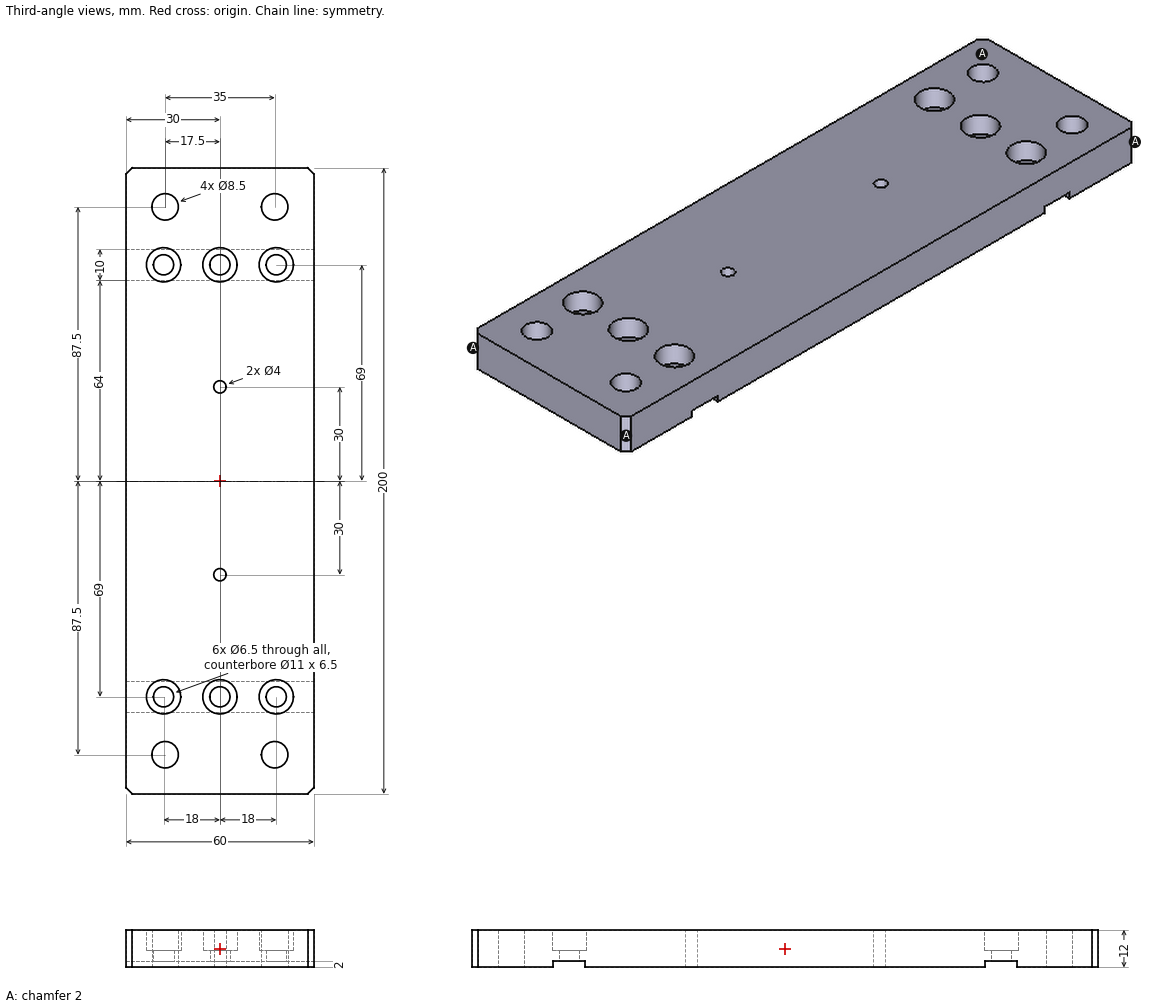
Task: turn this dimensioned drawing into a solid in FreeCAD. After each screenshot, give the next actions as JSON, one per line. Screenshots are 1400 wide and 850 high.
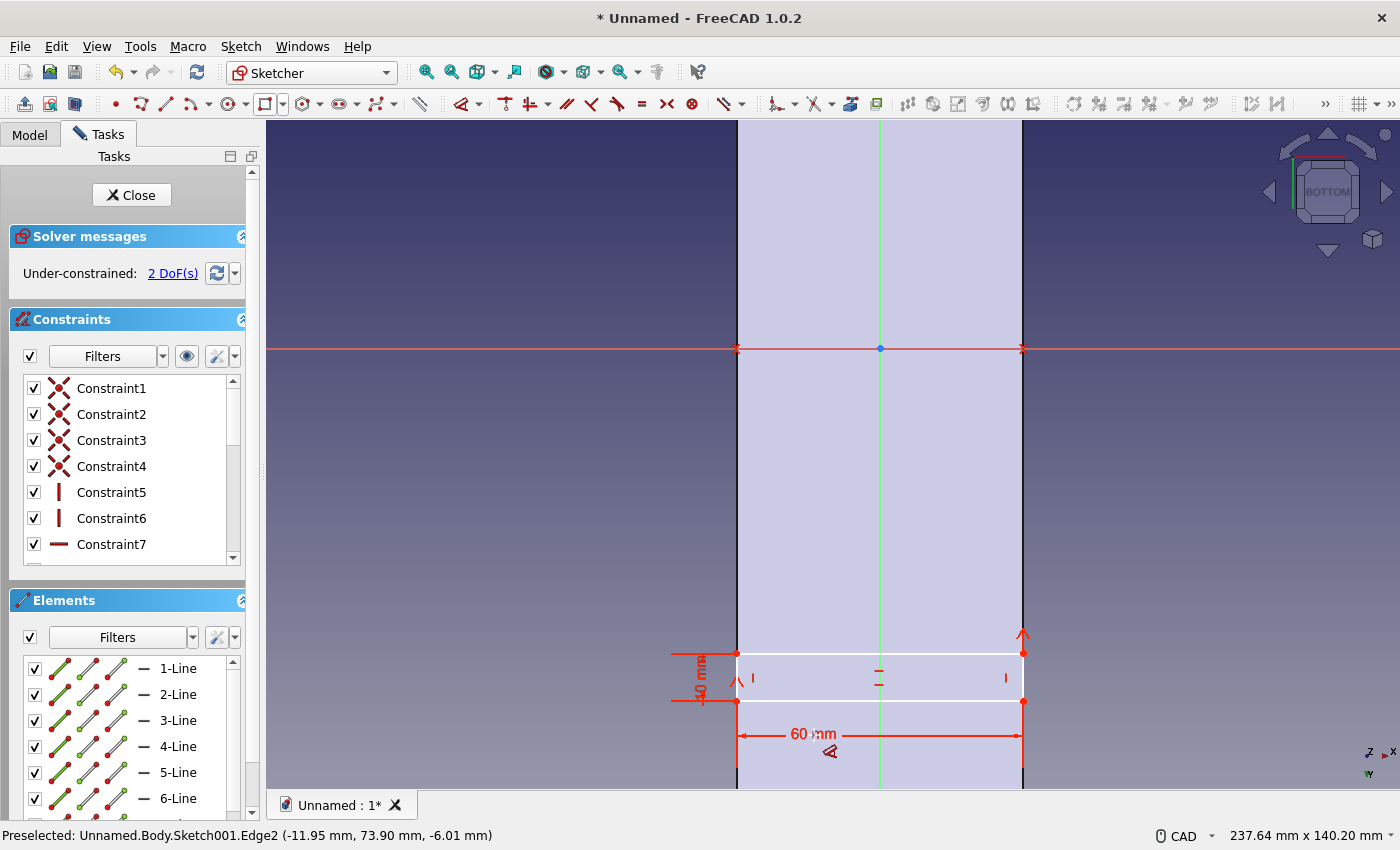
{"action": "left_click", "coordinate": [737, 654]}
{"action": "left_click", "coordinate": [808, 688]}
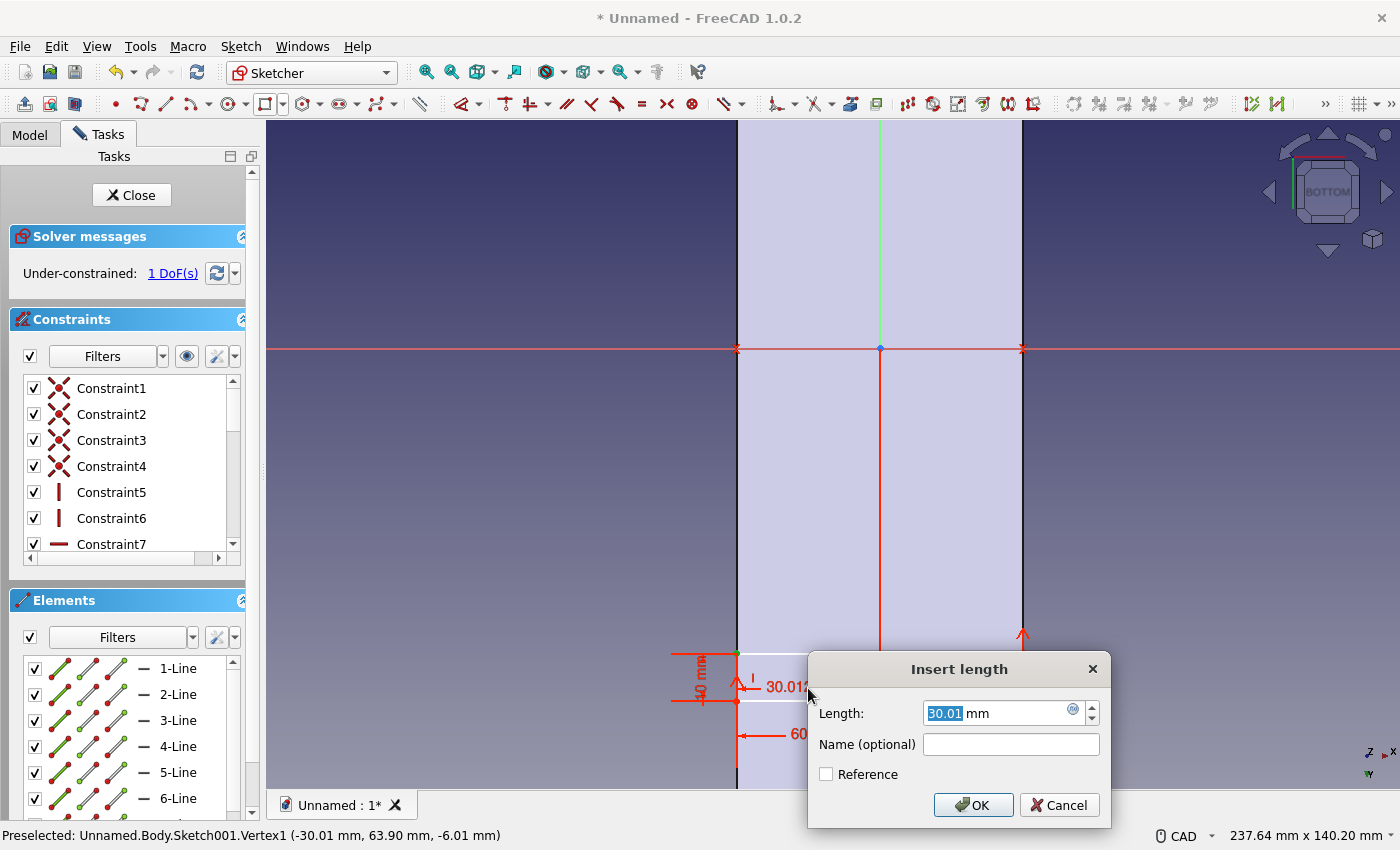
{"action": "type", "text": "30"}
{"action": "key", "text": "Return"}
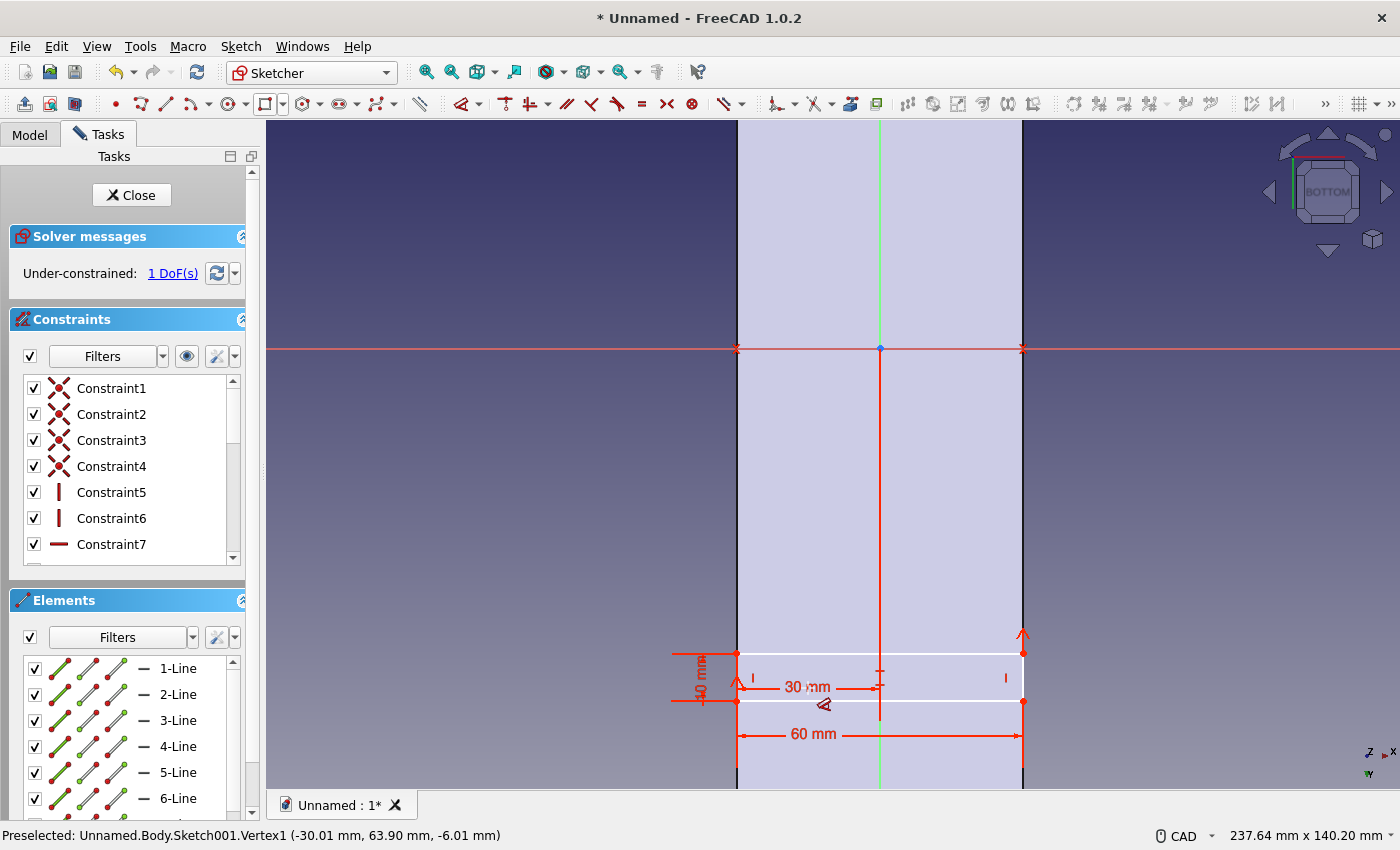
{"action": "left_click", "coordinate": [737, 654]}
{"action": "left_click", "coordinate": [703, 501]}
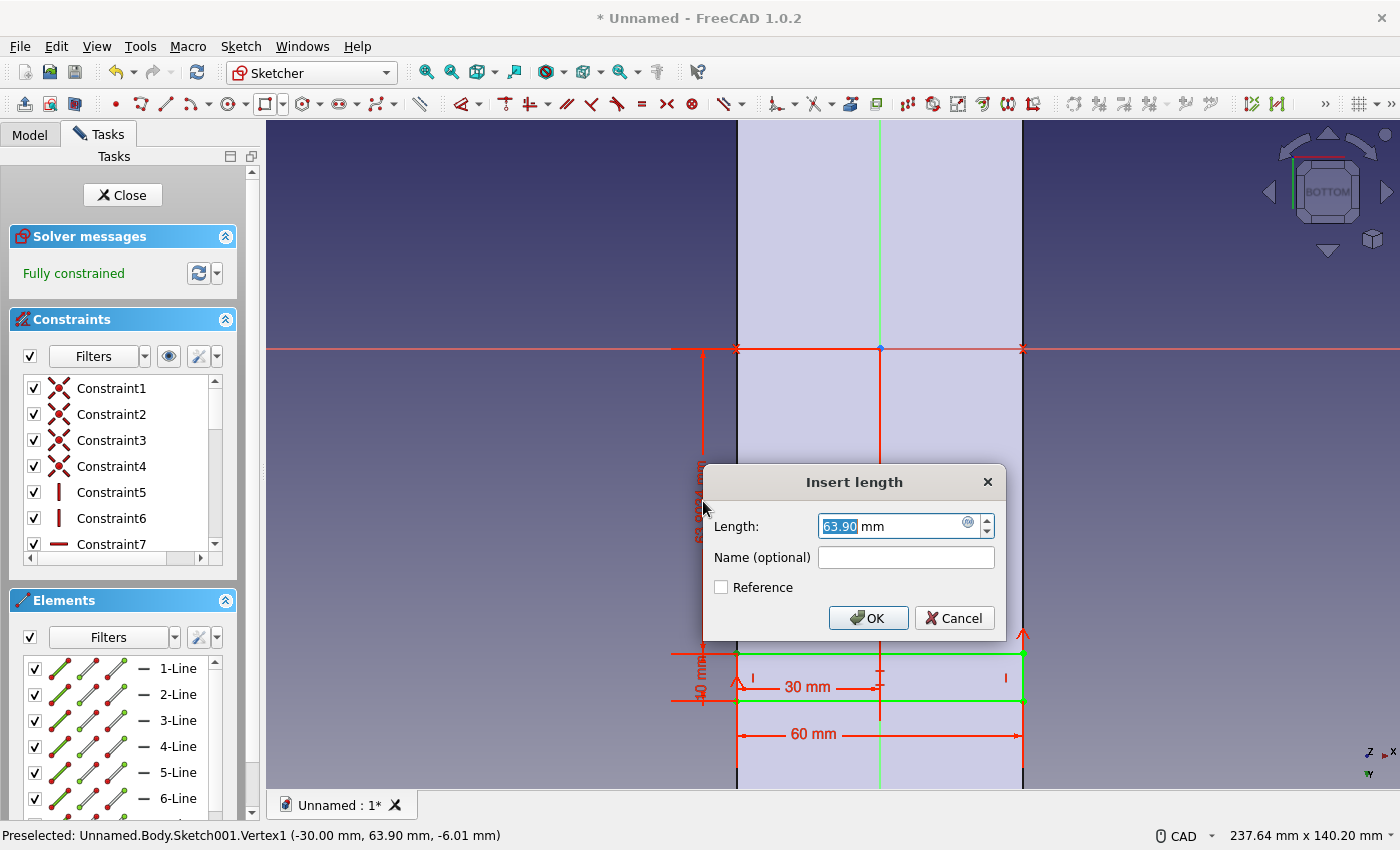
{"action": "type", "text": "64"}
{"action": "key", "text": "Return"}
{"action": "key", "text": "Escape"}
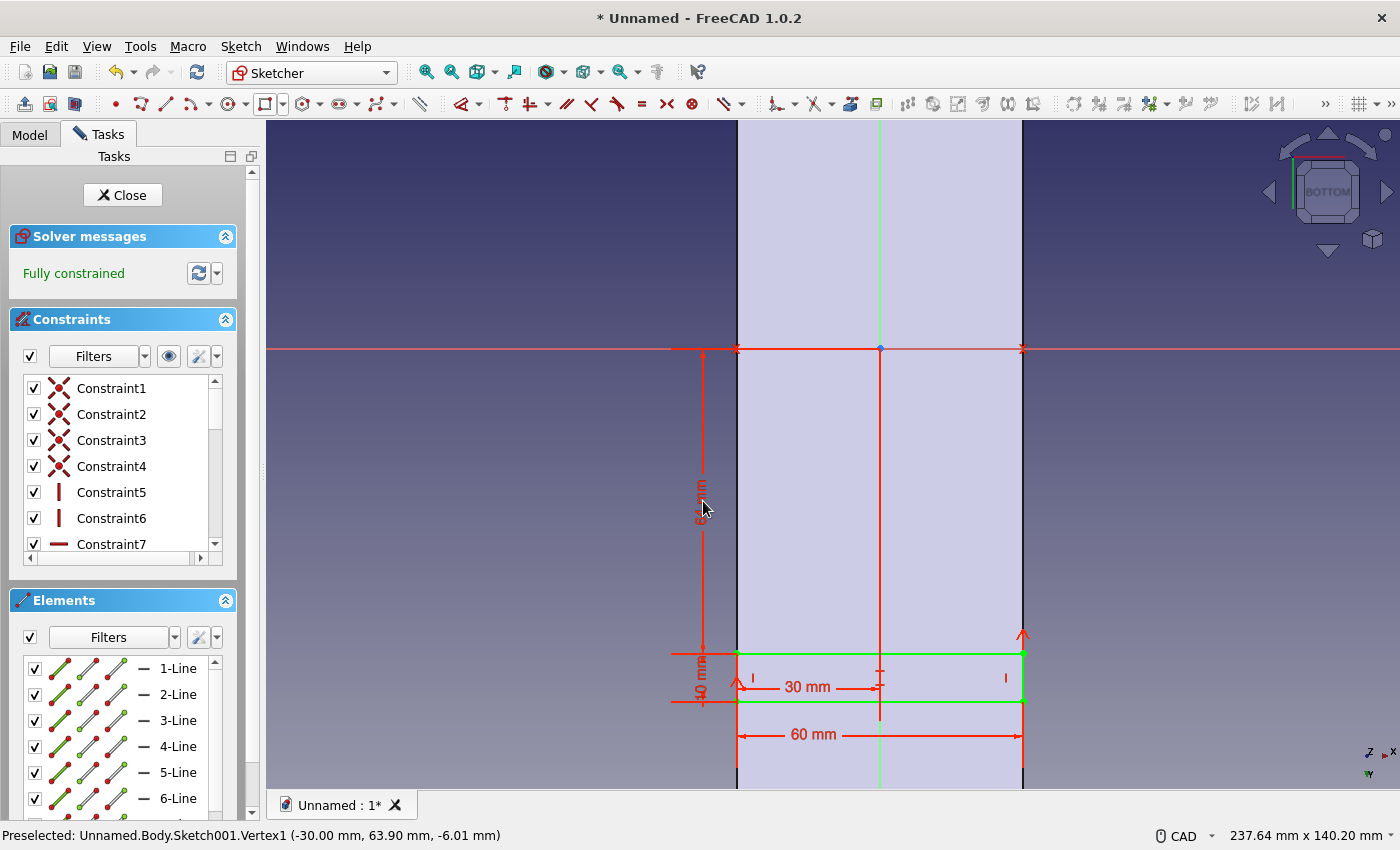
{"action": "left_click", "coordinate": [123, 195]}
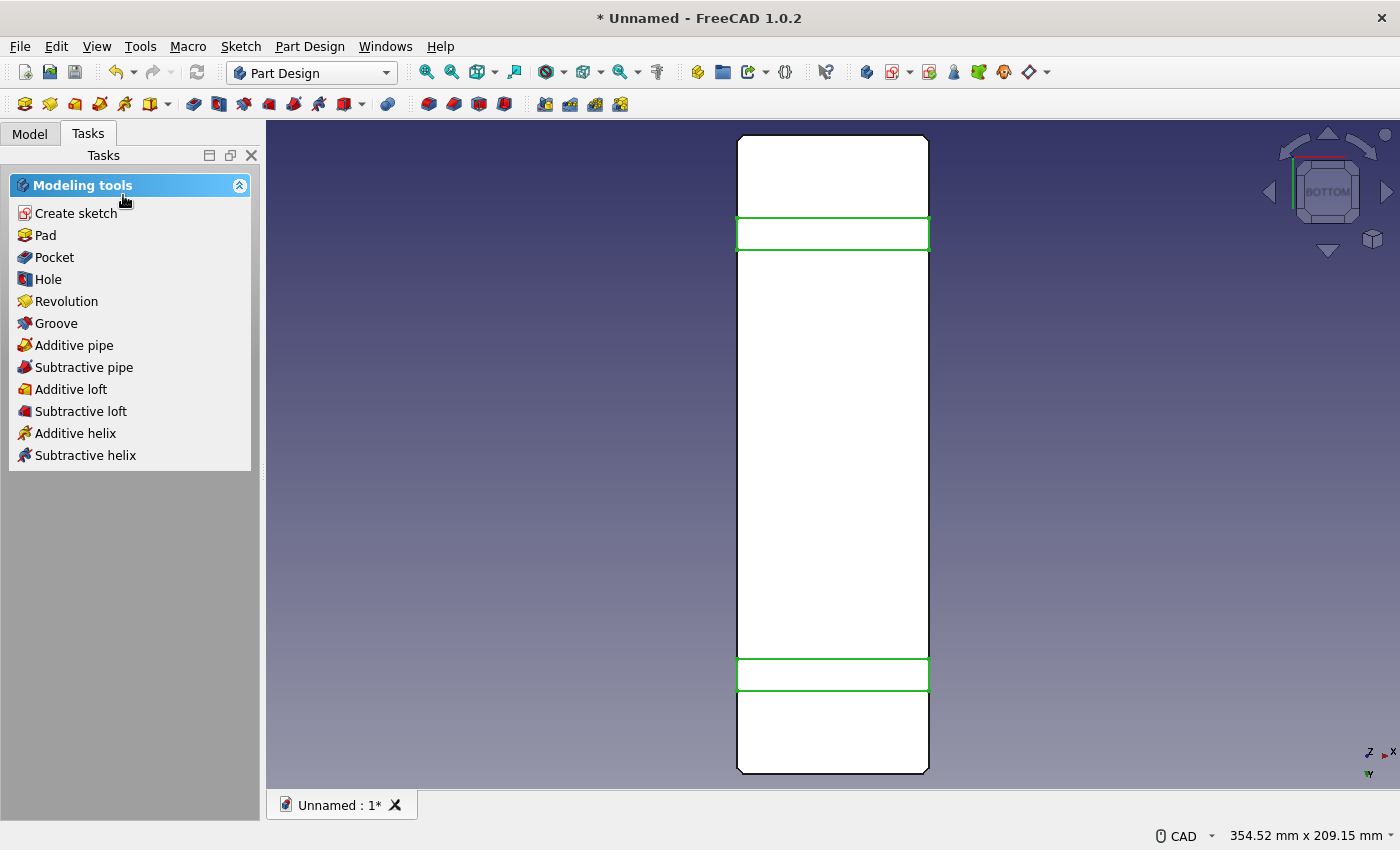
{"action": "left_click", "coordinate": [194, 104]}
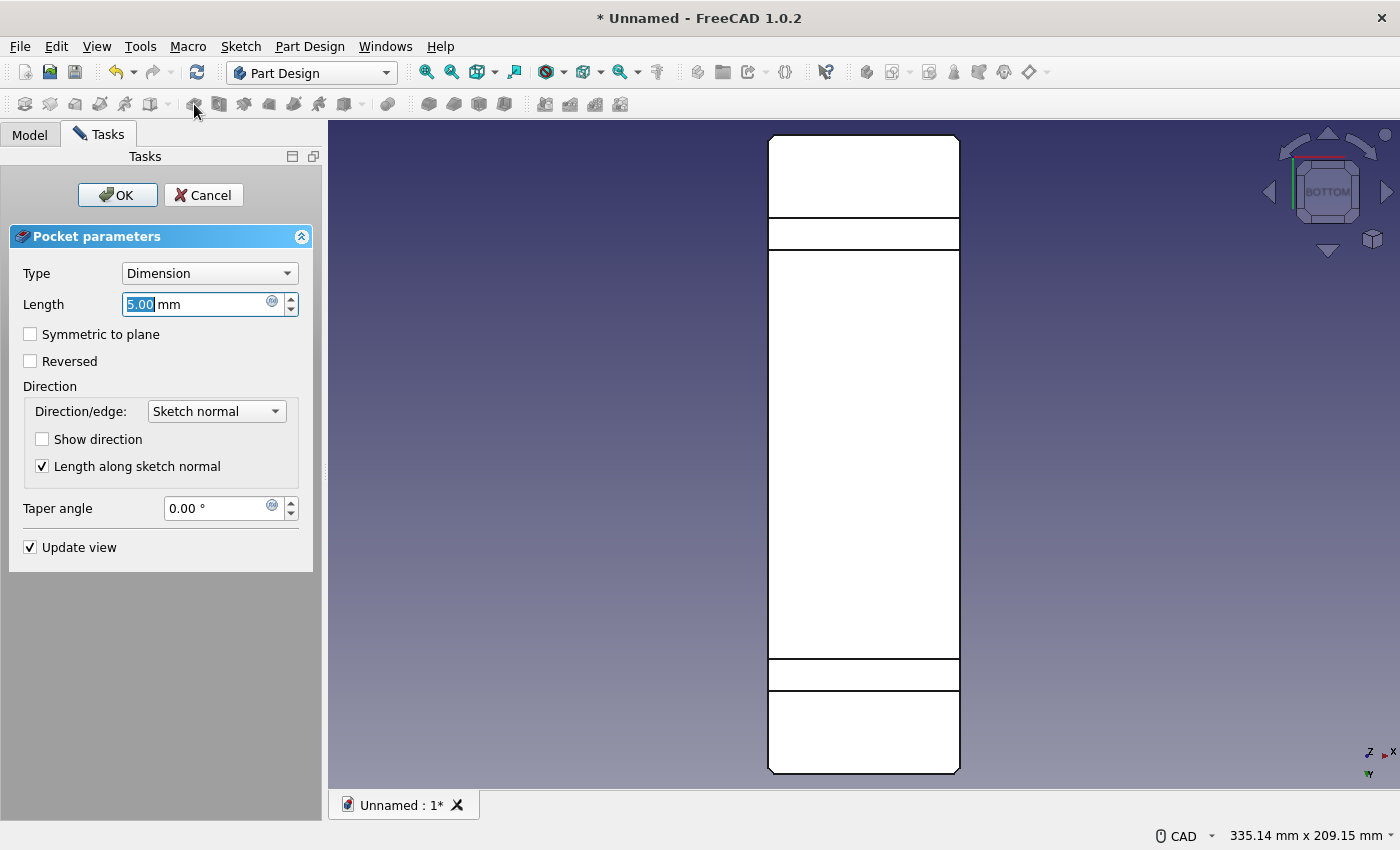
{"action": "type", "text": "2"}
{"action": "key", "text": "Tab"}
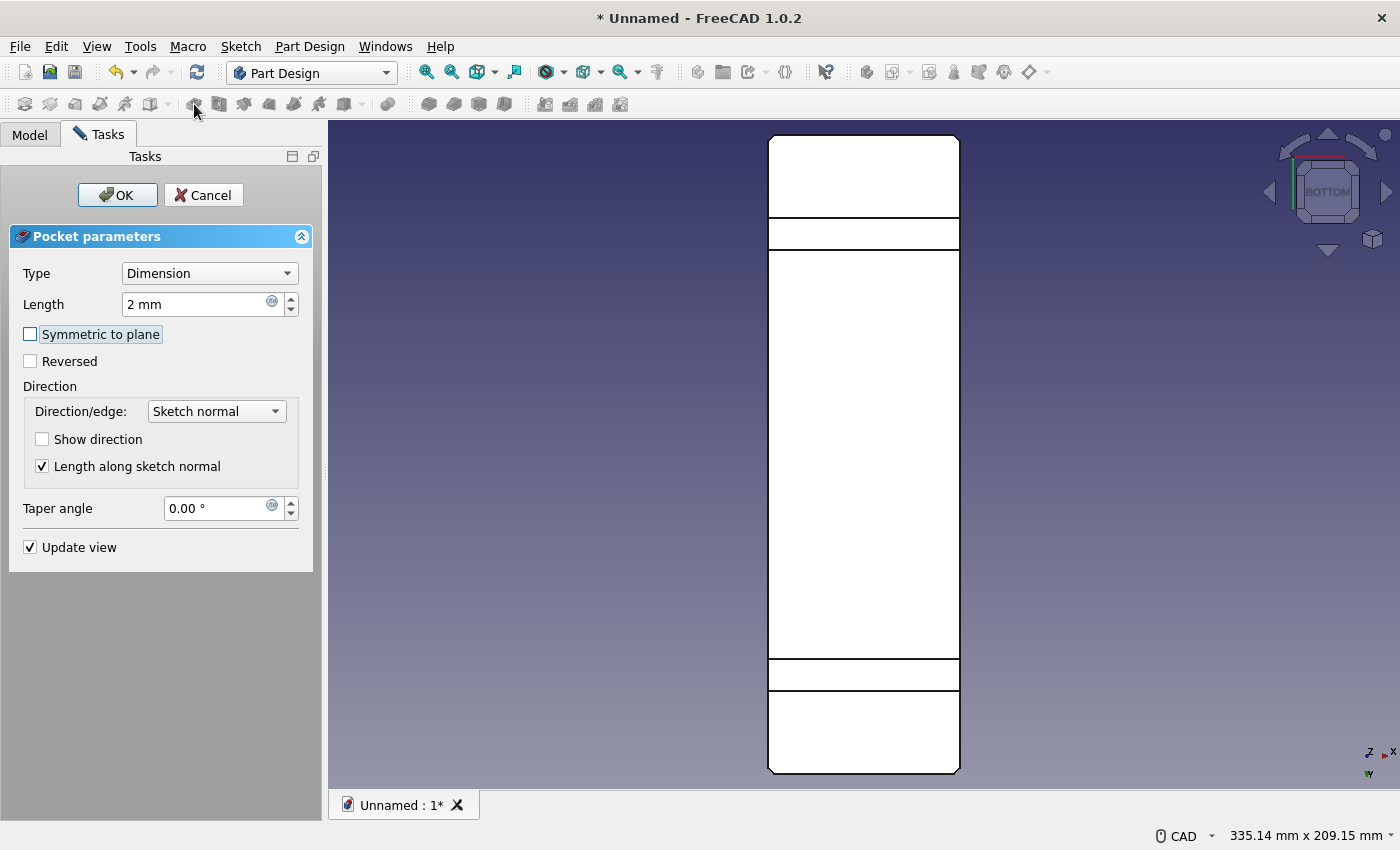
{"action": "left_click", "coordinate": [118, 195]}